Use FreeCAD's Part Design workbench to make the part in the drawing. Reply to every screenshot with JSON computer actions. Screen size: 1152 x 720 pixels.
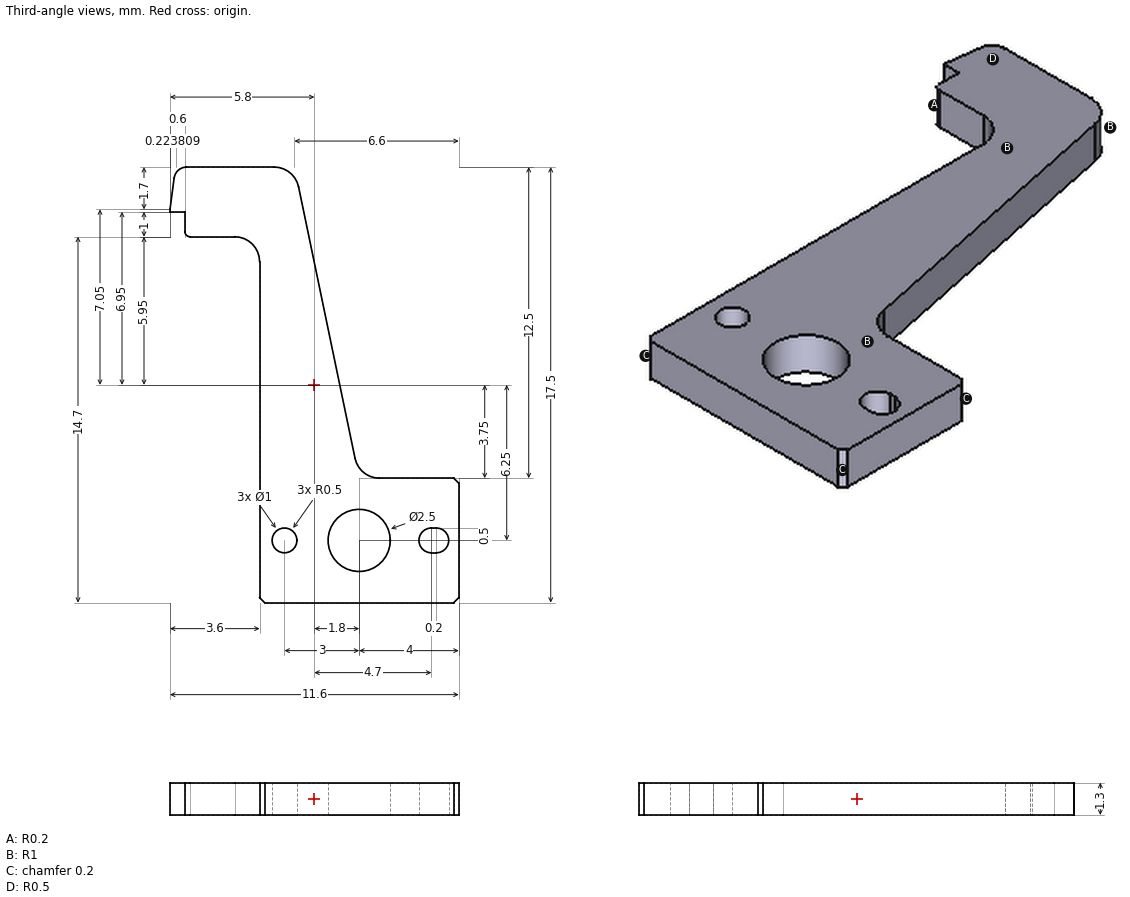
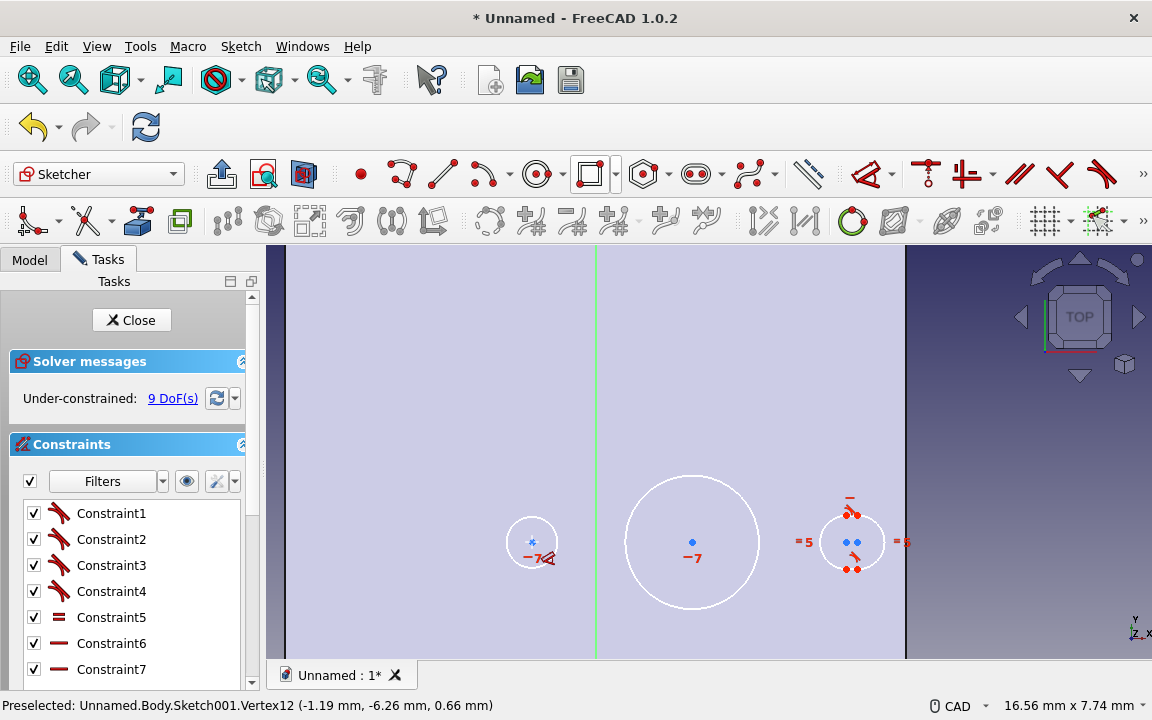
{"action": "scroll", "coordinate": [825, 527], "scroll_direction": "up", "scroll_amount": 2}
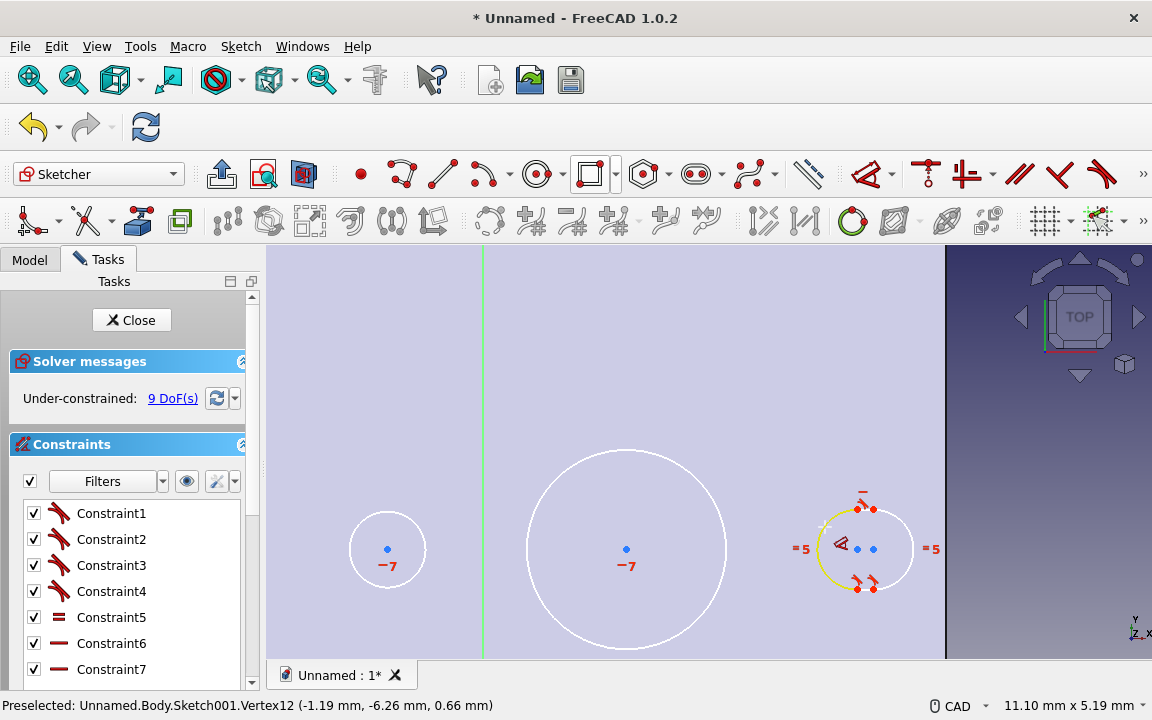
{"action": "left_click", "coordinate": [825, 526]}
{"action": "left_click", "coordinate": [799, 507]}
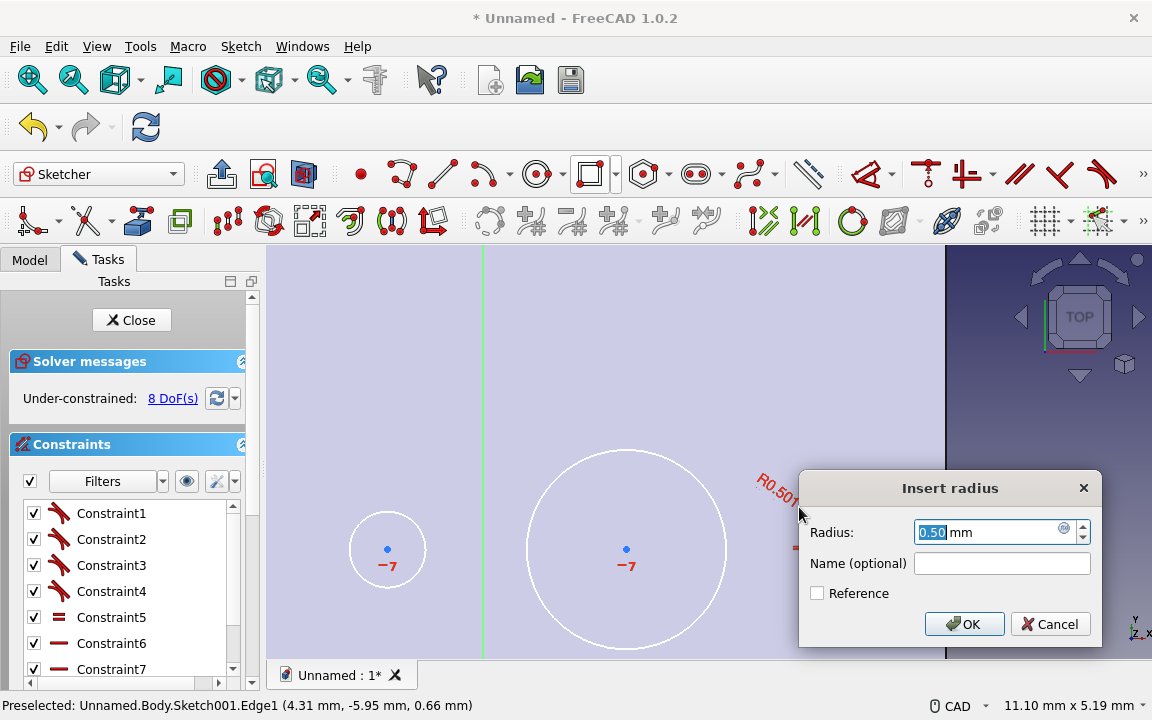
{"action": "type", "text": "0.5"}
{"action": "key", "text": "Return"}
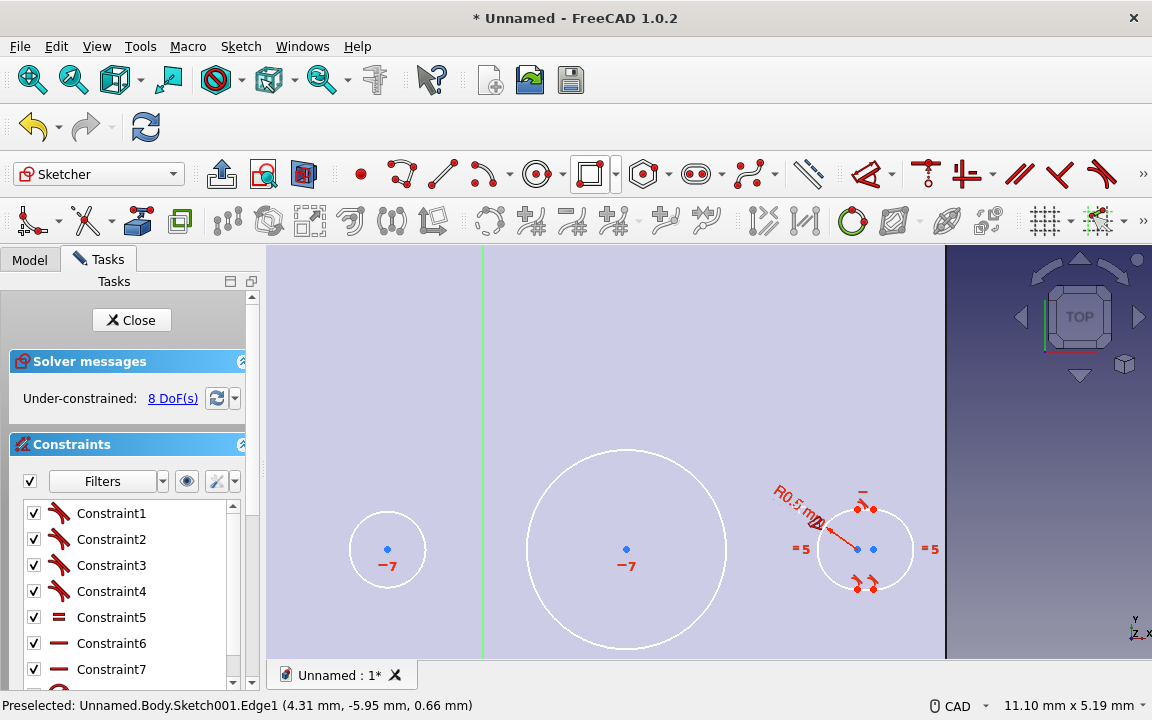
{"action": "left_click", "coordinate": [697, 479]}
{"action": "left_click", "coordinate": [720, 456]}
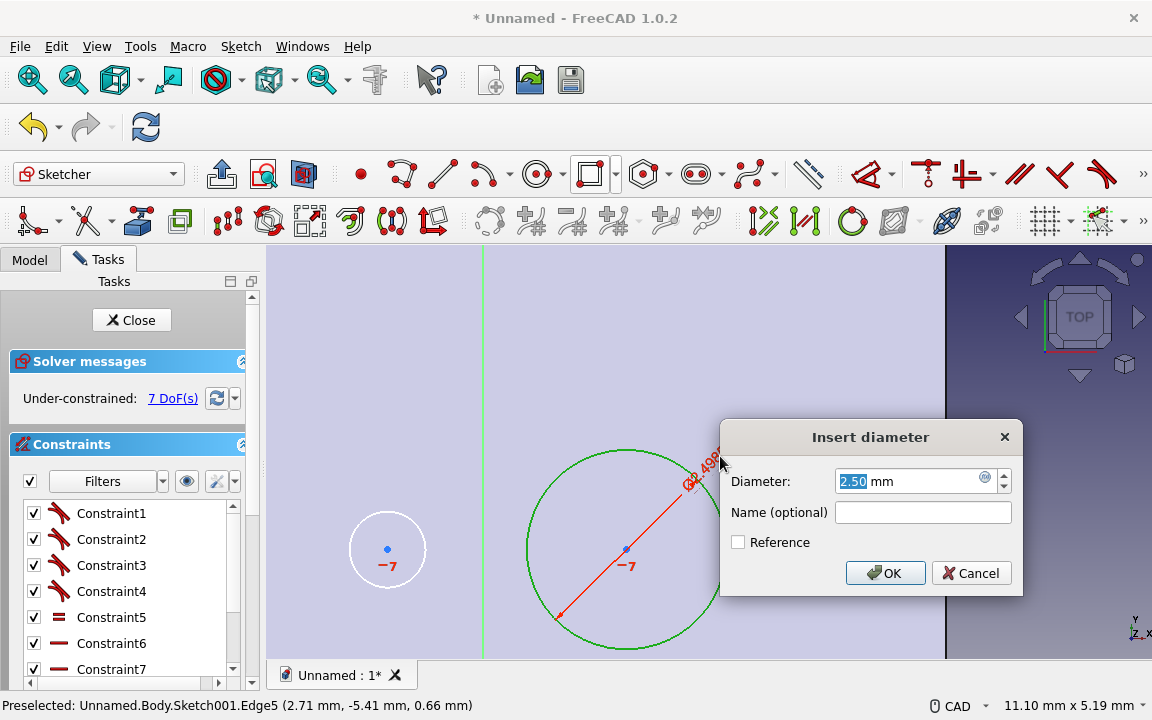
{"action": "type", "text": "2.5"}
{"action": "key", "text": "Return"}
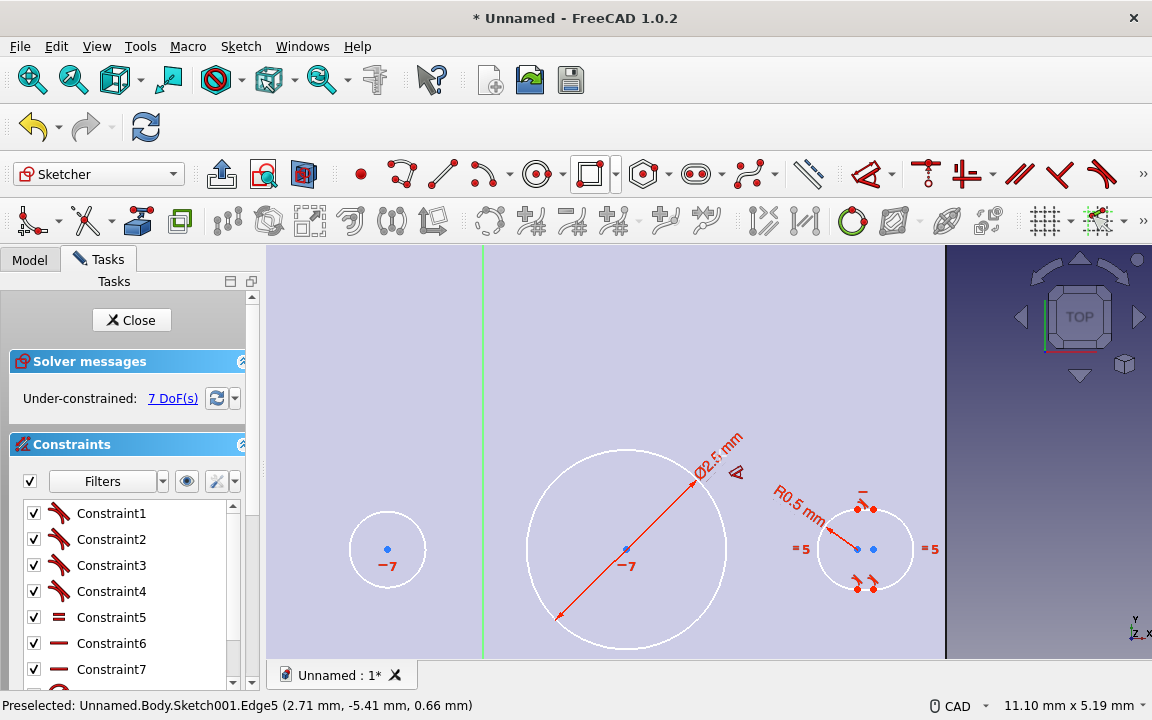
{"action": "left_click", "coordinate": [414, 523]}
{"action": "left_click", "coordinate": [437, 500]}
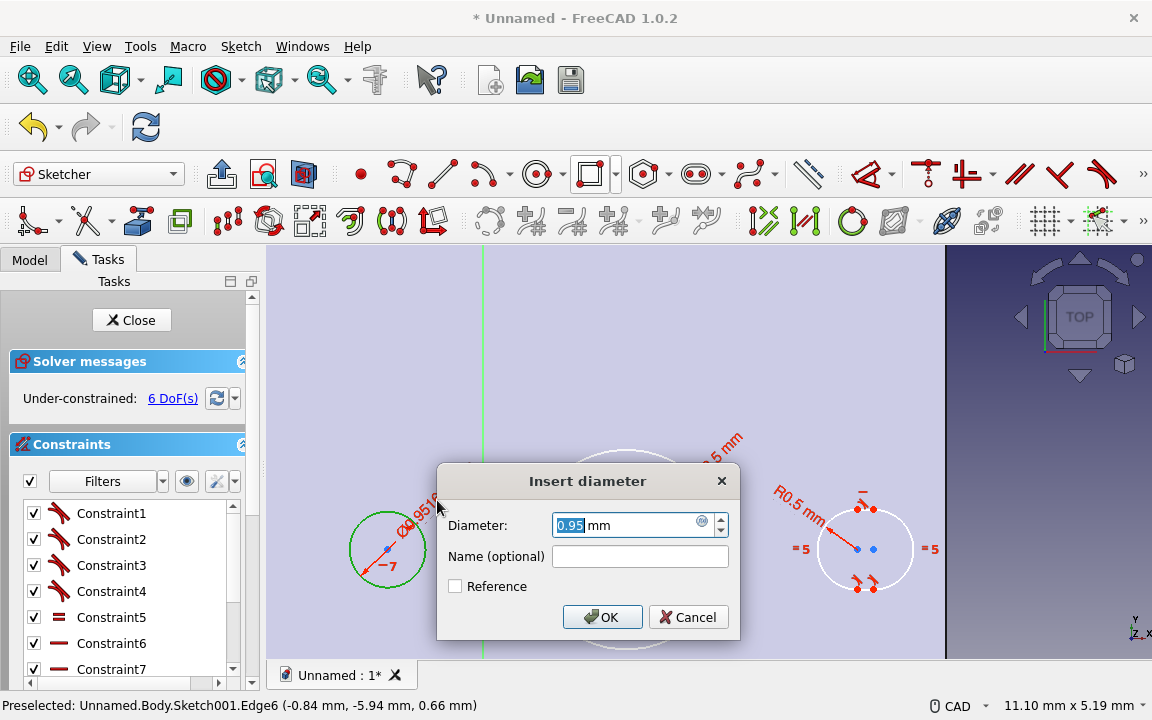
{"action": "type", "text": "1"}
{"action": "key", "text": "Return"}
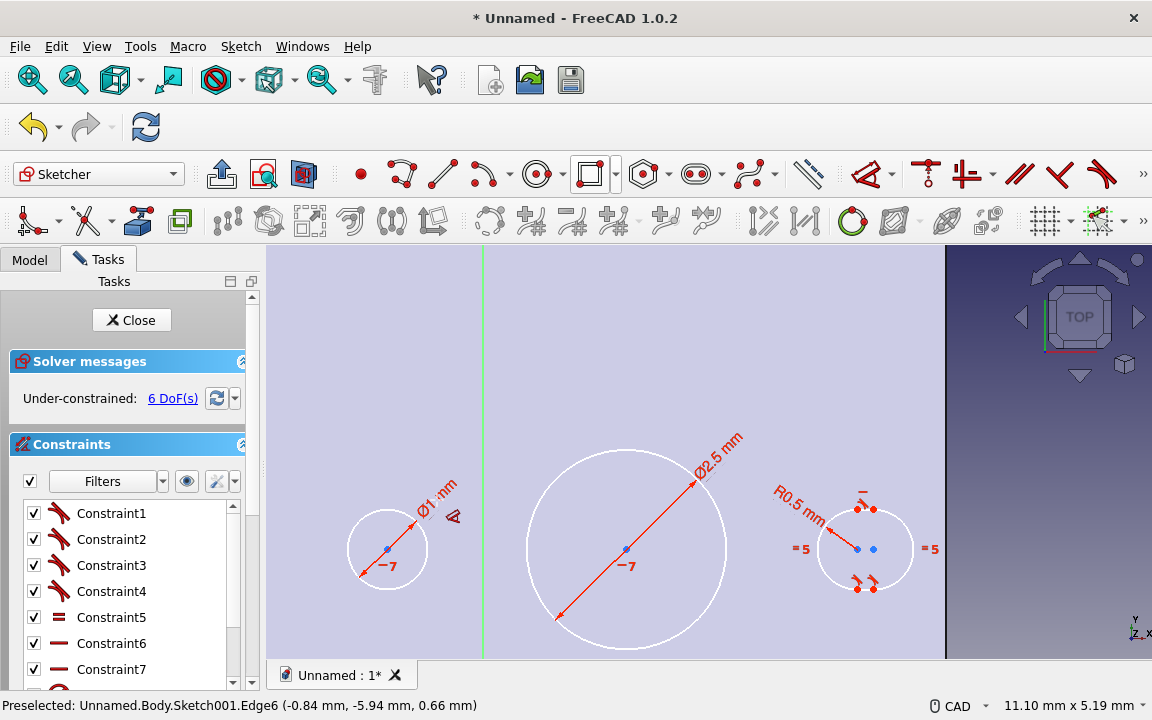
{"action": "left_click", "coordinate": [626, 550]}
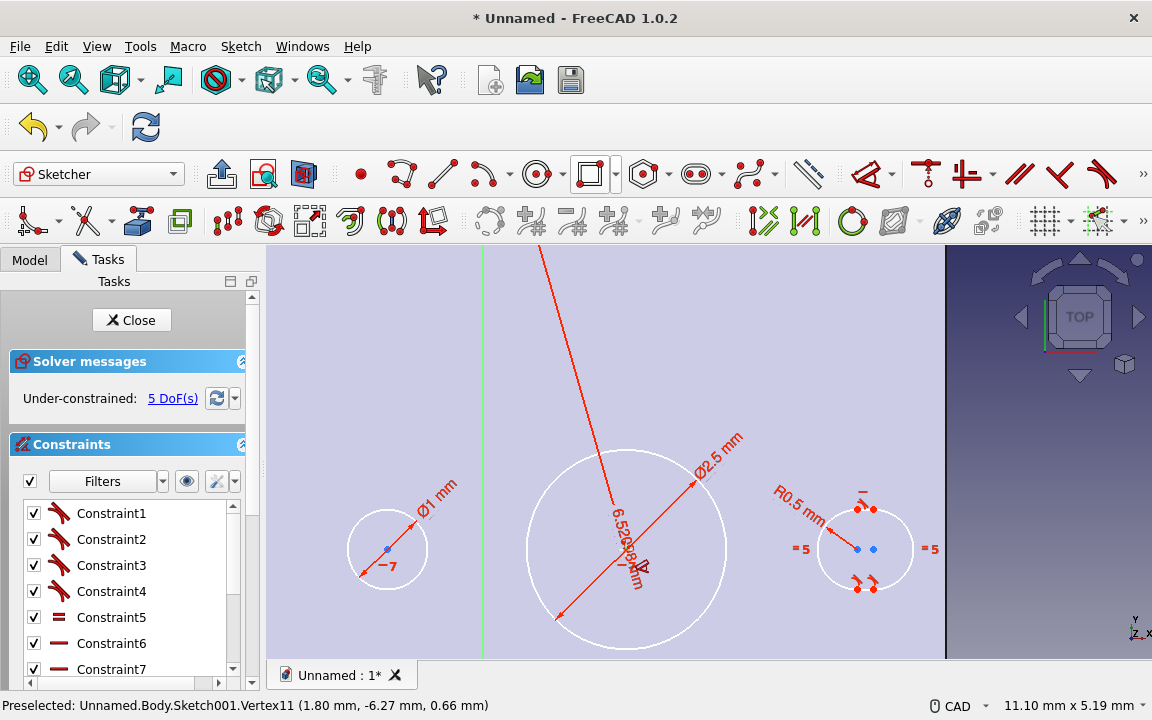
{"action": "left_click", "coordinate": [388, 550]}
{"action": "left_click", "coordinate": [507, 584]}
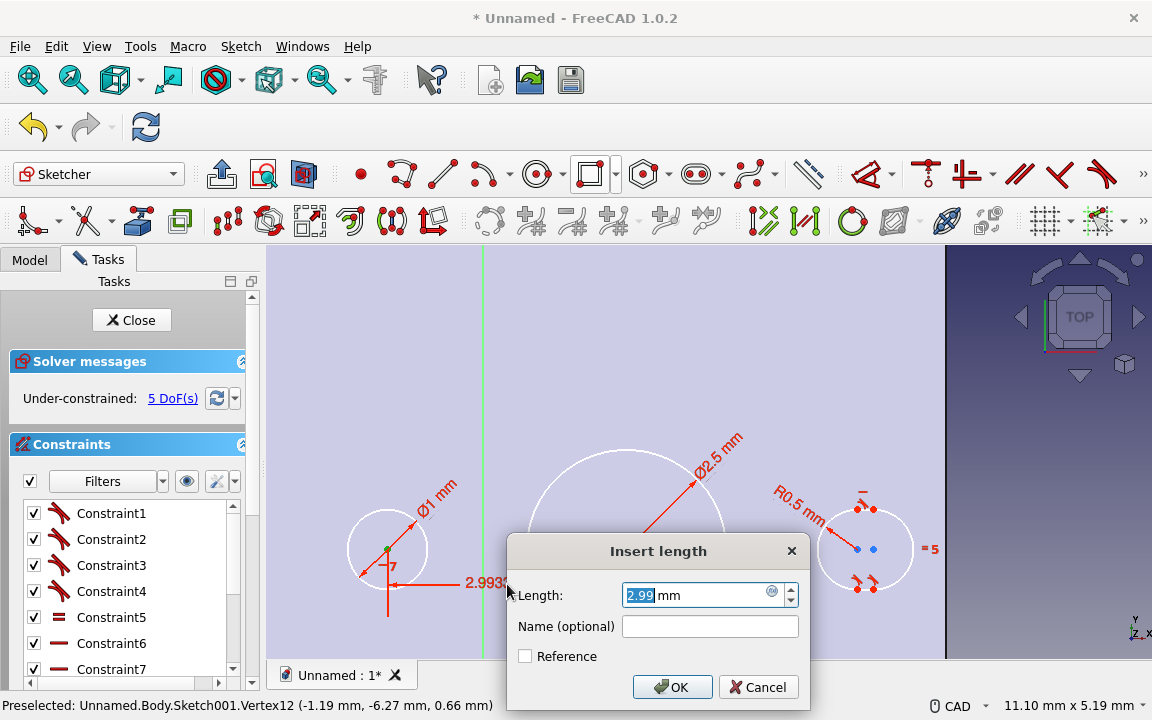
{"action": "type", "text": "3"}
{"action": "key", "text": "Return"}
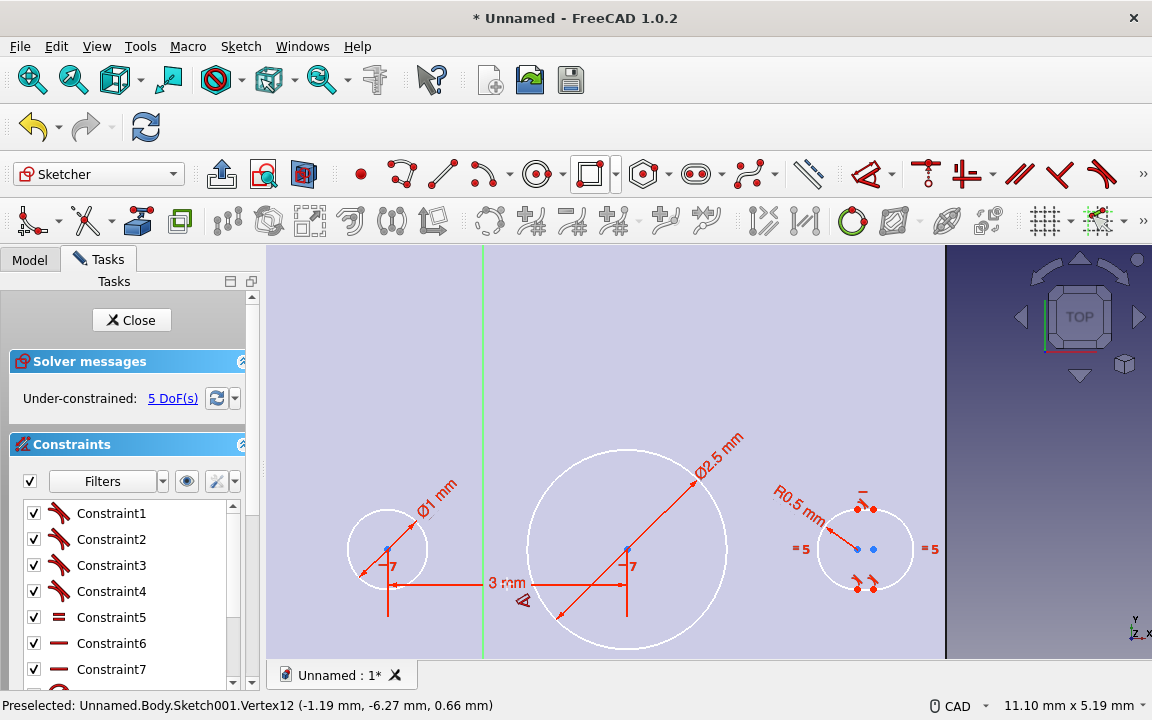
{"action": "scroll", "coordinate": [865, 510], "scroll_direction": "up", "scroll_amount": 5}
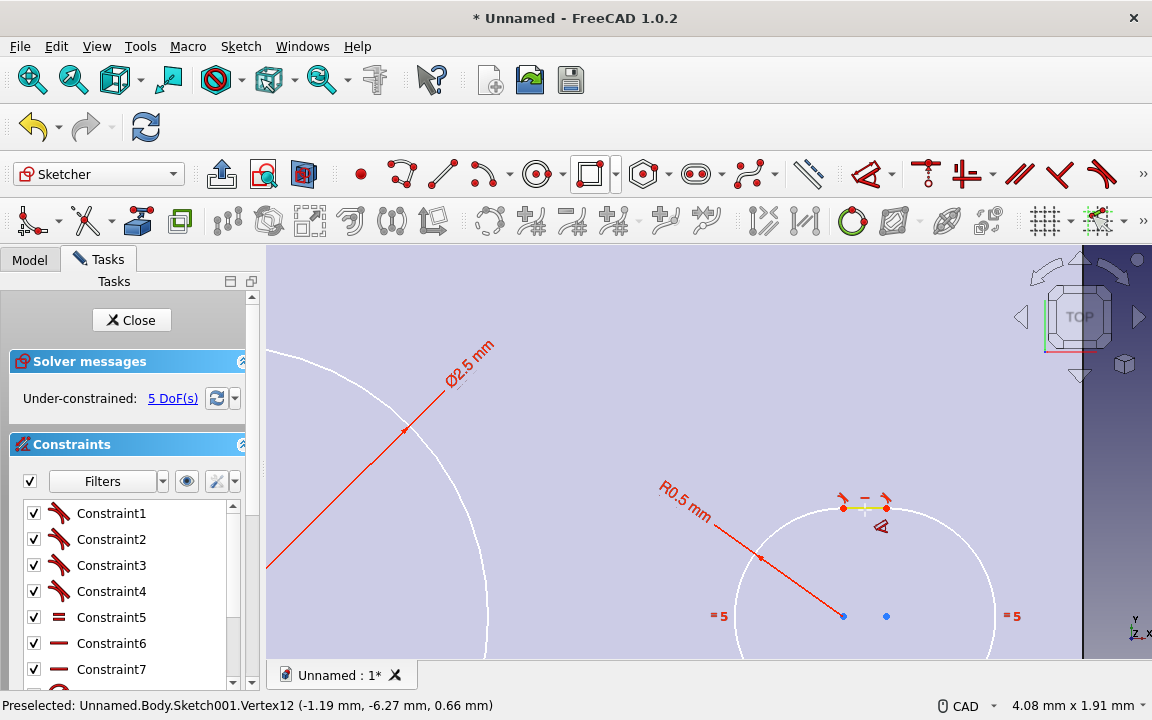
{"action": "left_click", "coordinate": [865, 508]}
{"action": "left_click", "coordinate": [865, 542]}